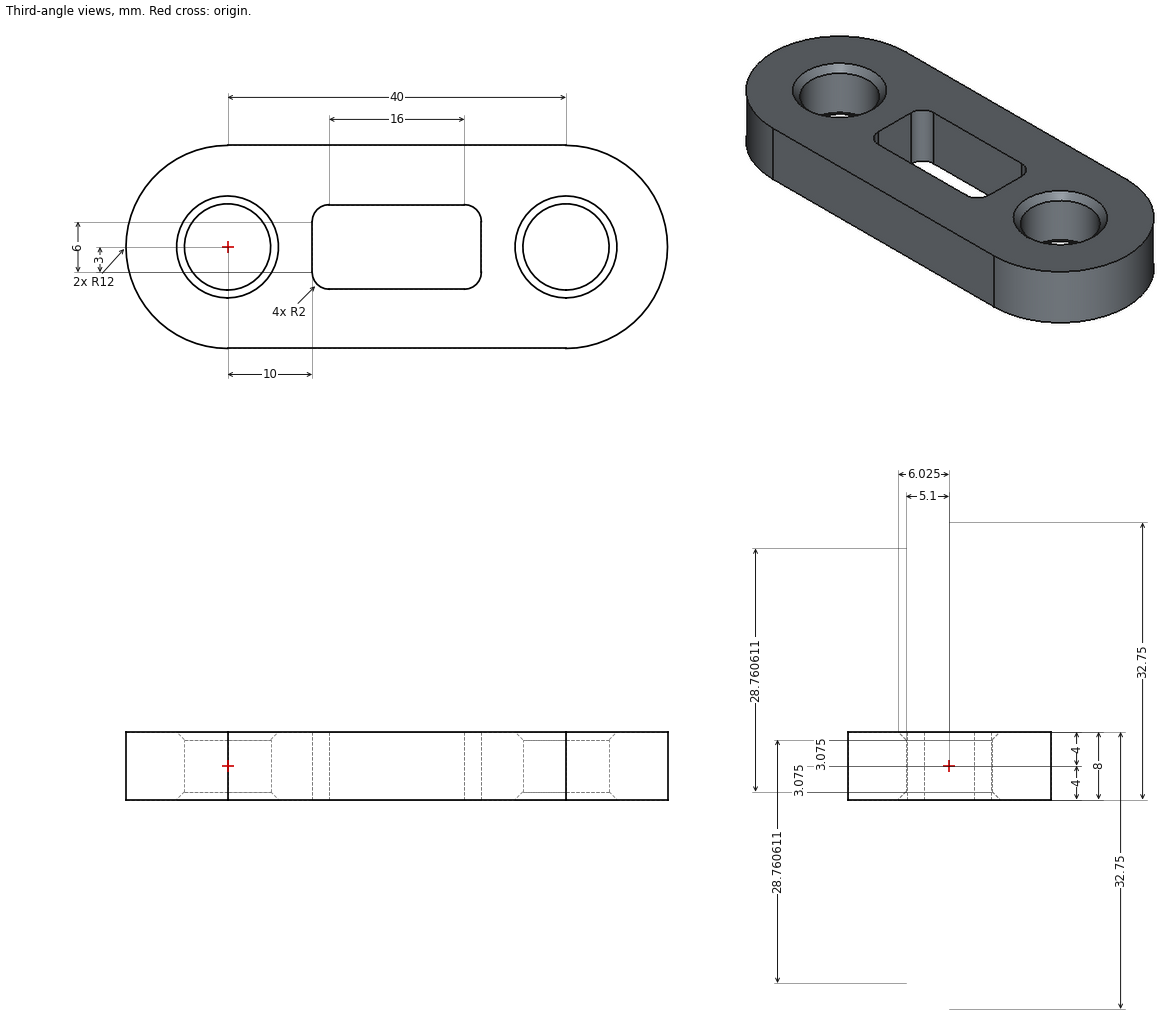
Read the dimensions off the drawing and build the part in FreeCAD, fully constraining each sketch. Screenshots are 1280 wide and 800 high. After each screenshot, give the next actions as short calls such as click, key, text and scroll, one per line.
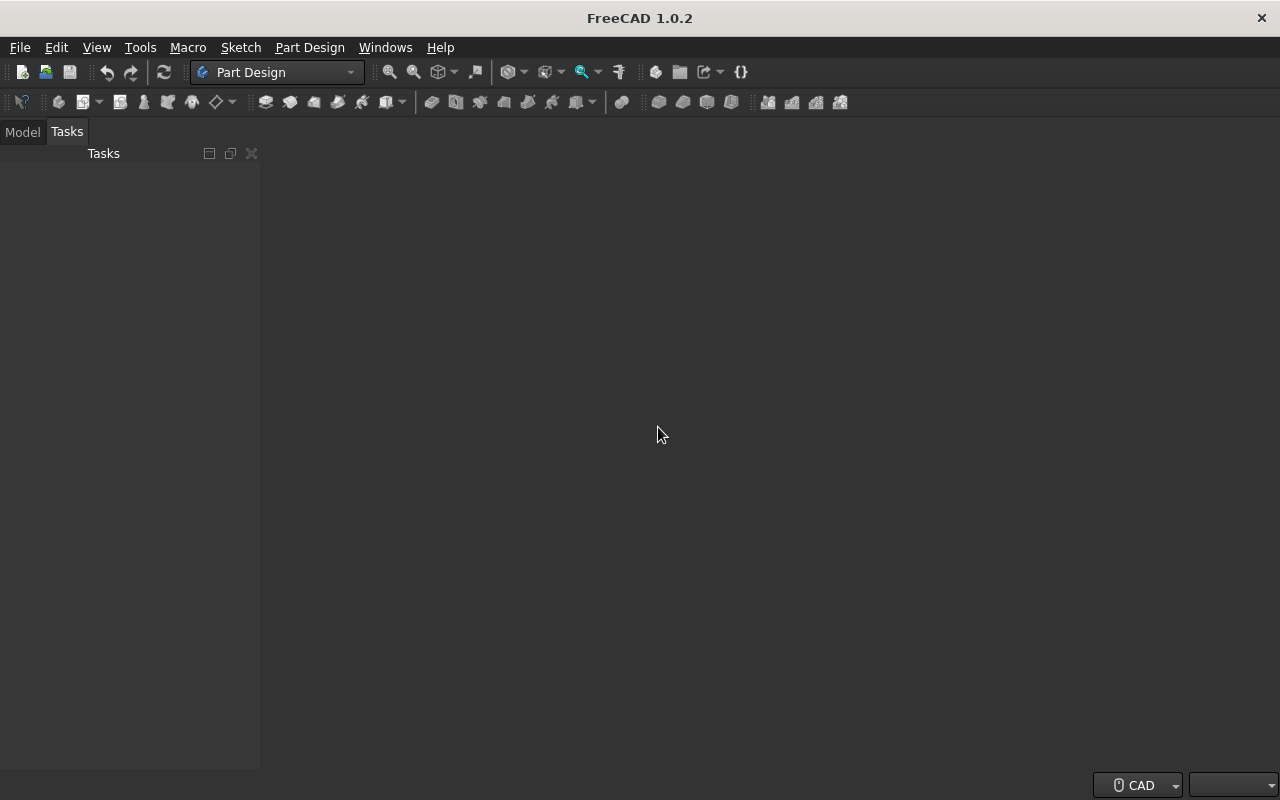
key(ctrl+n)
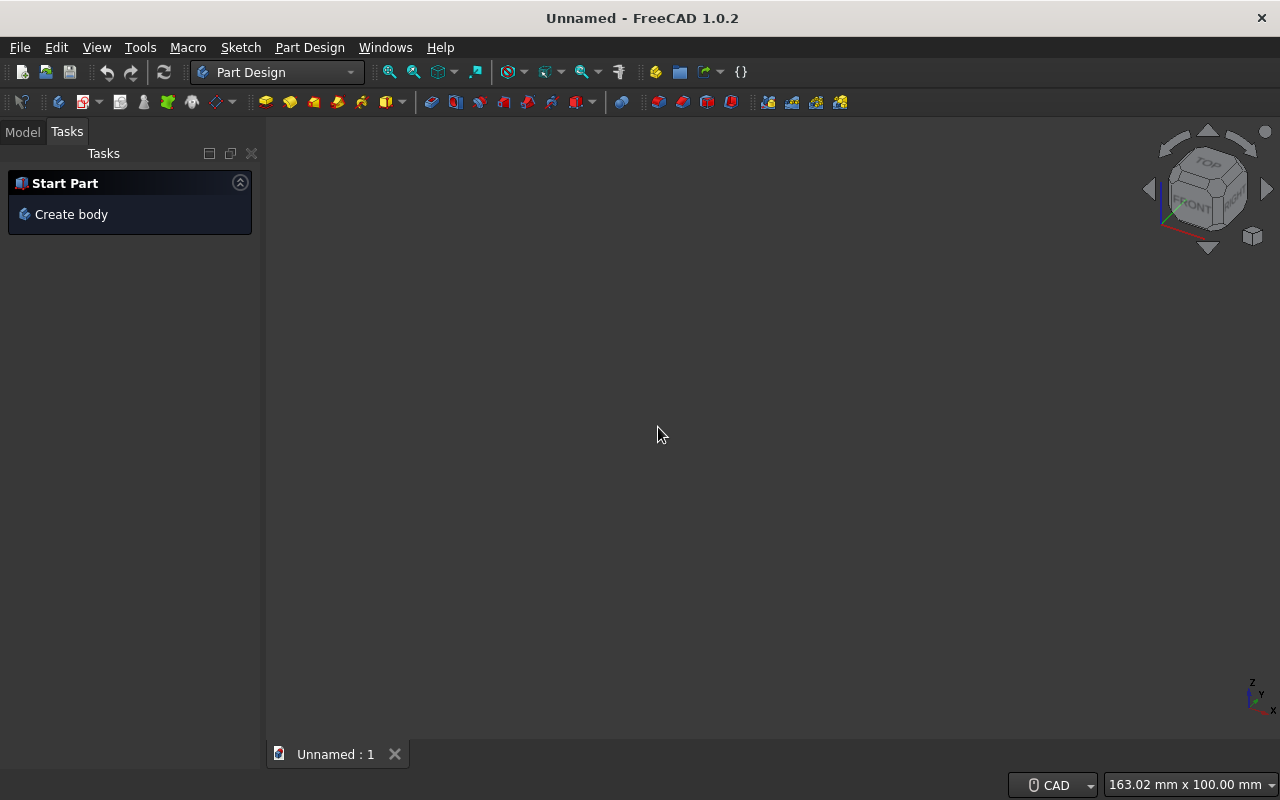
click(84, 102)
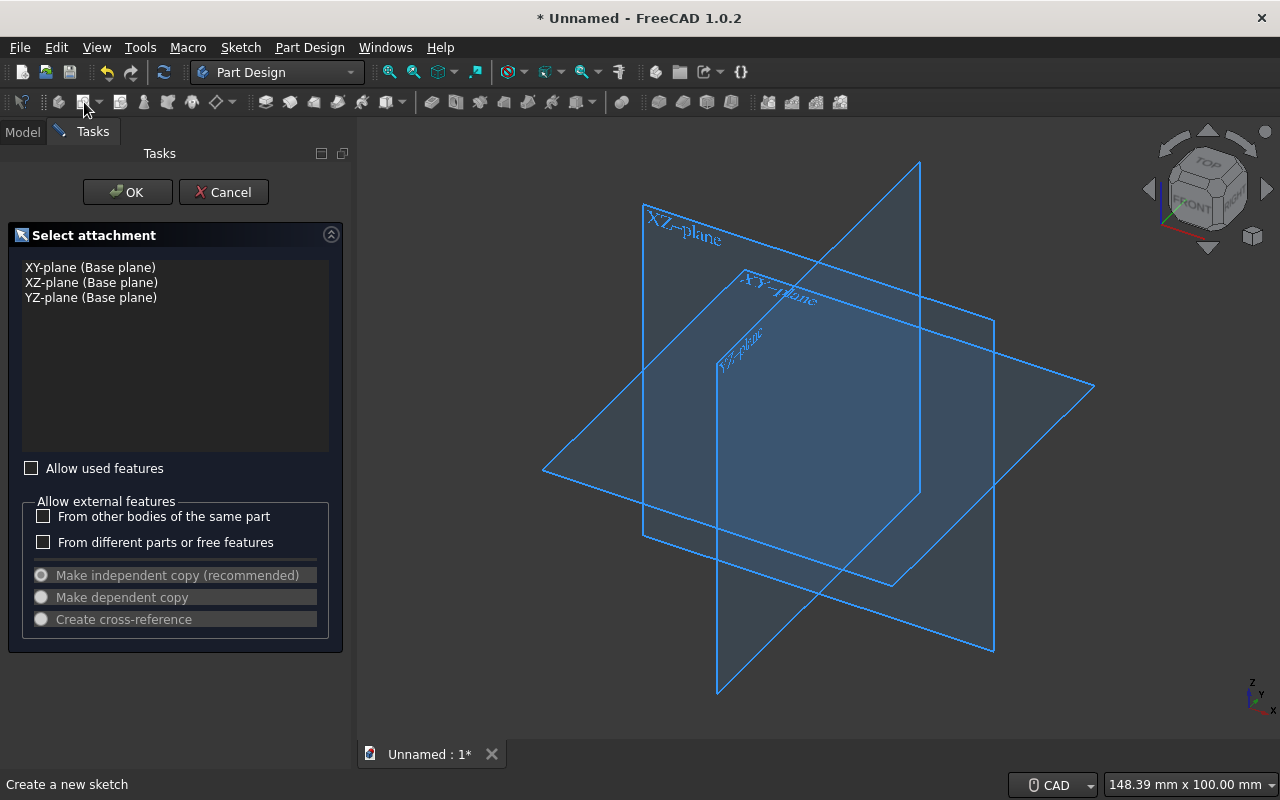
click(82, 268)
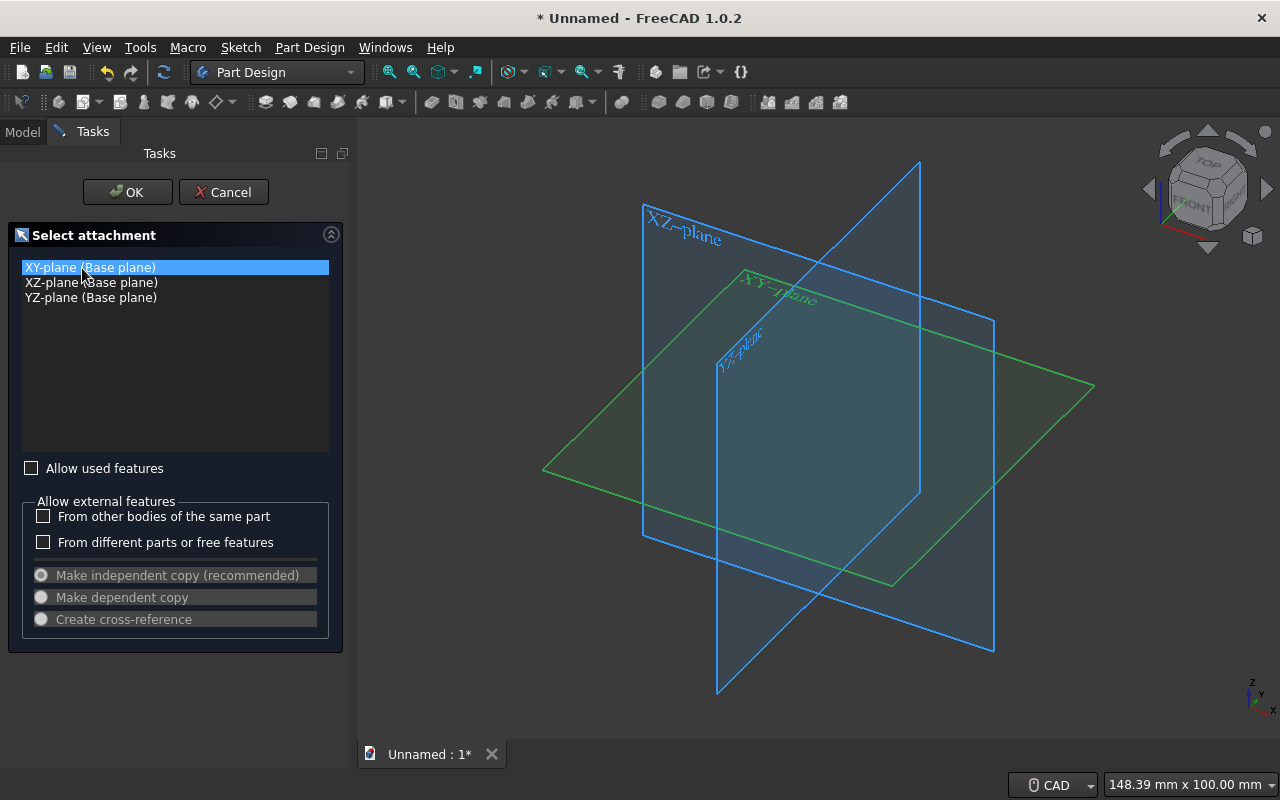
click(128, 192)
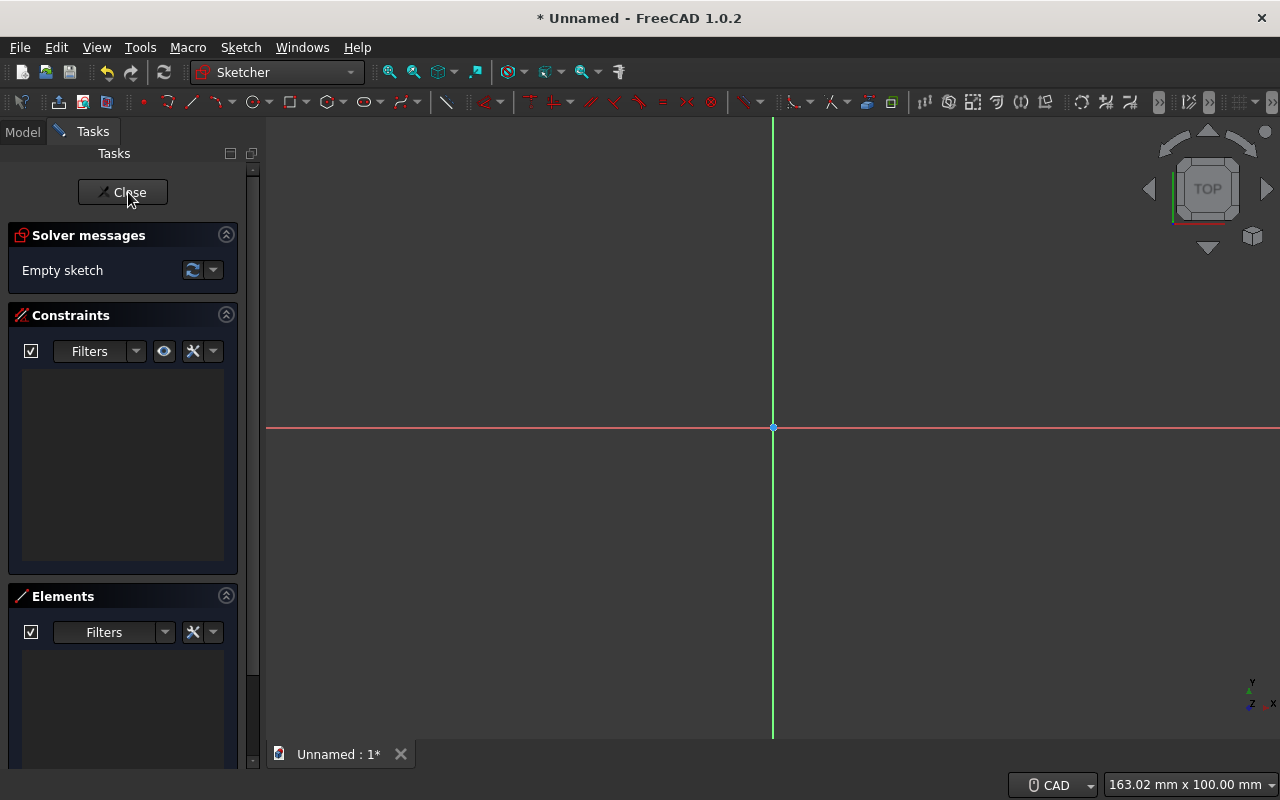
scroll(1115, 428, up, 2)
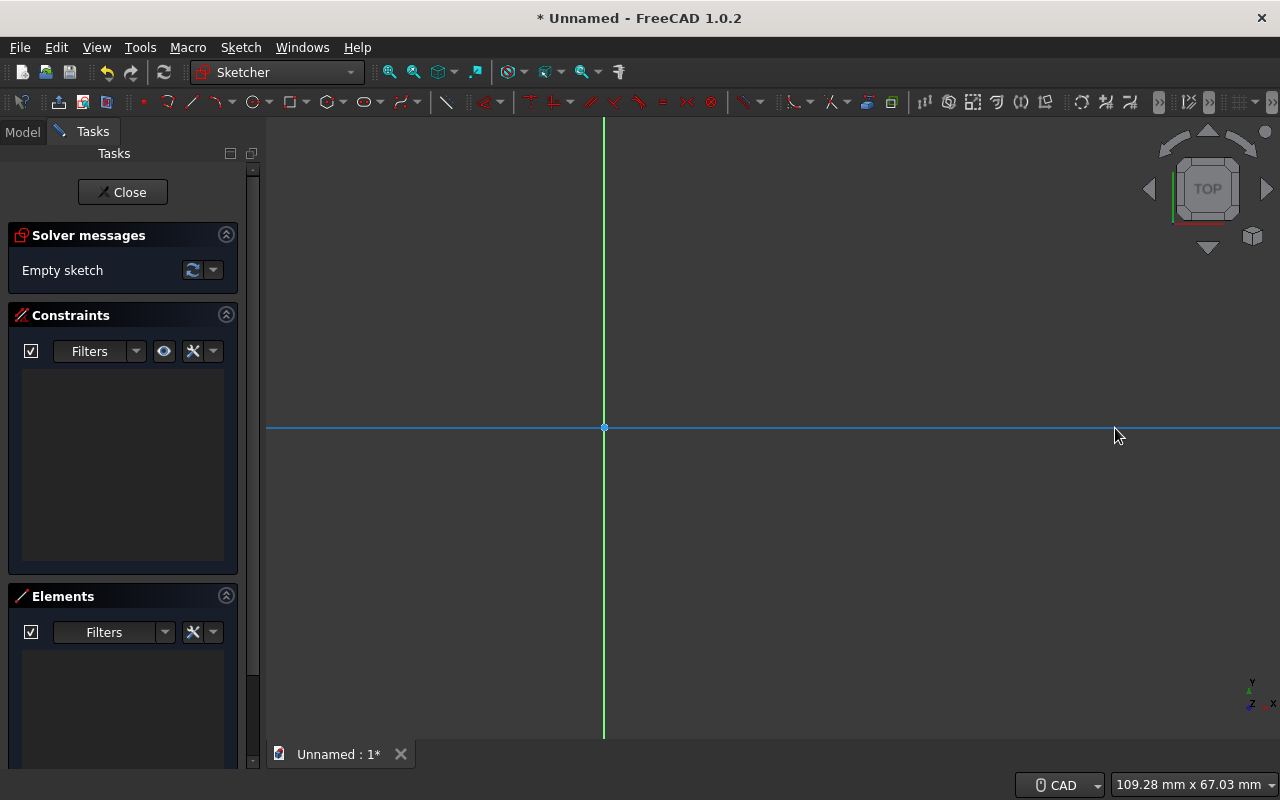
key(g)
key(s)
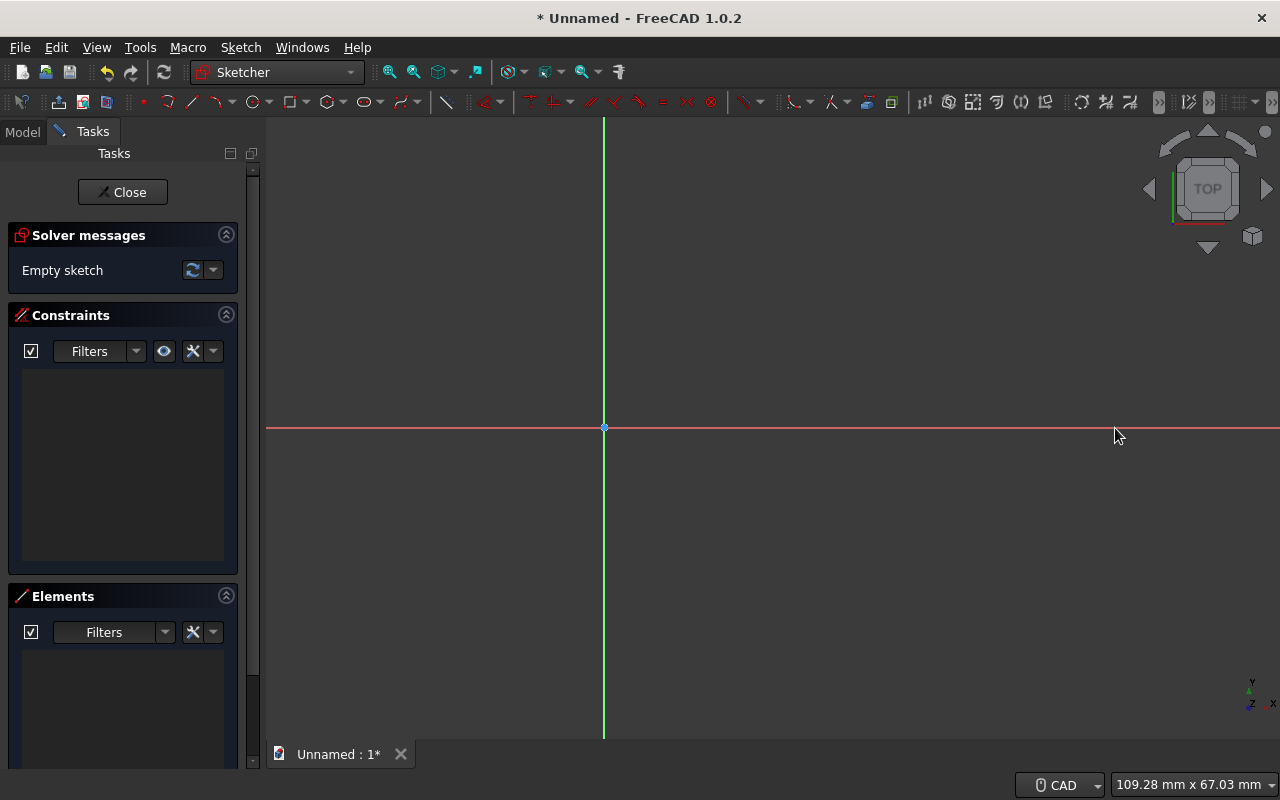
click(604, 428)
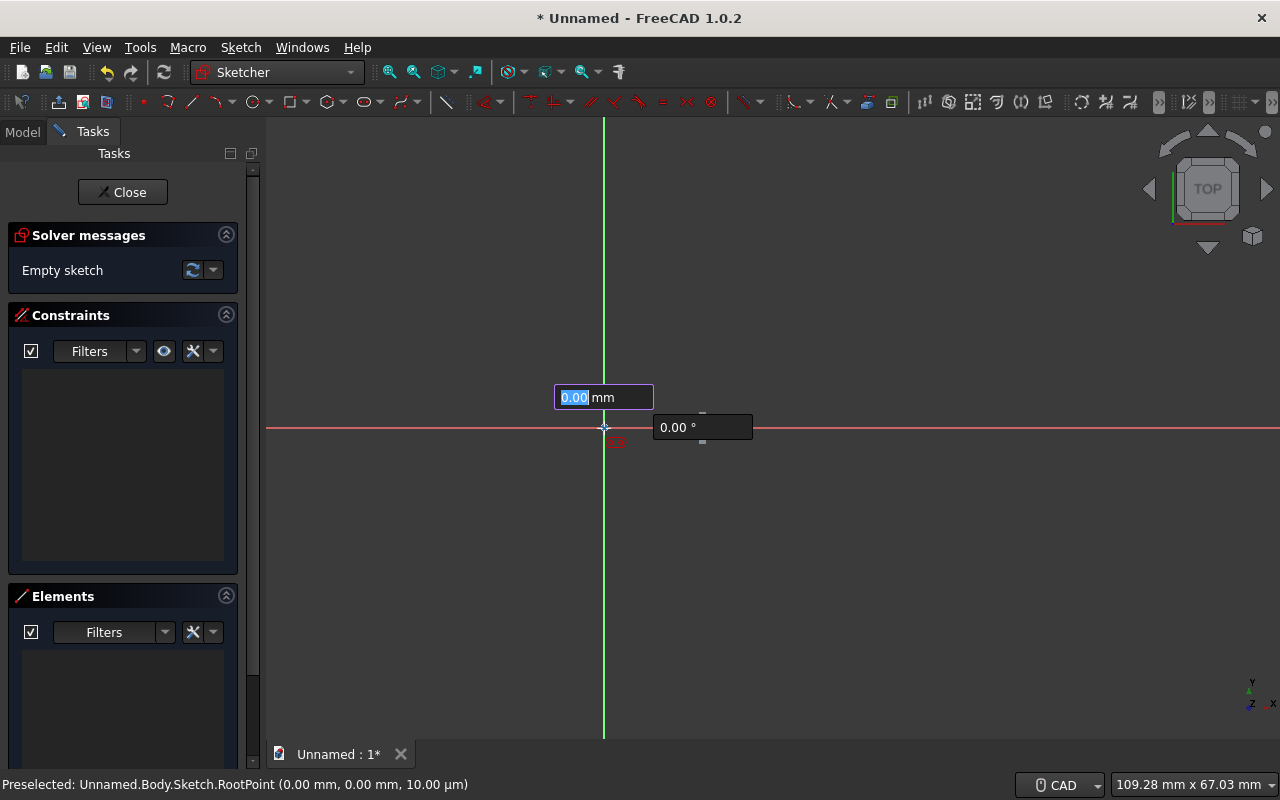
click(976, 419)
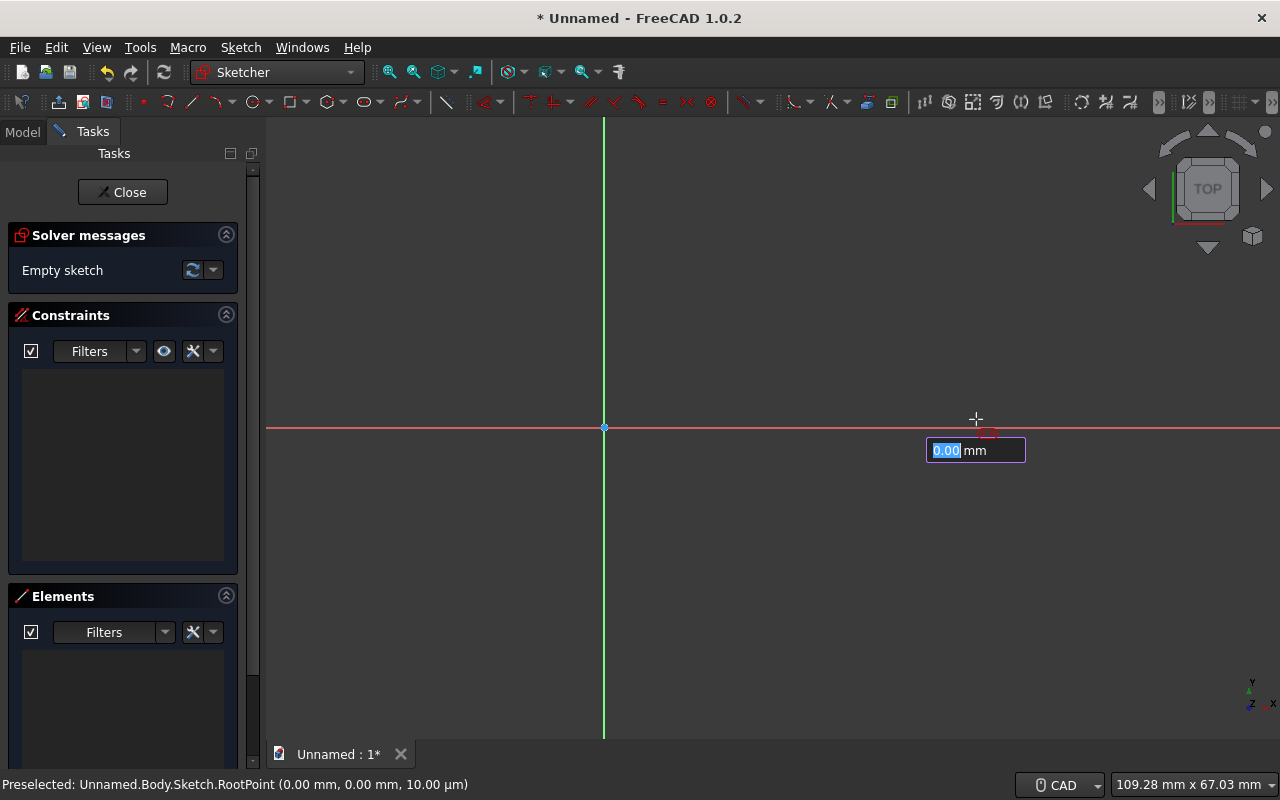
click(790, 316)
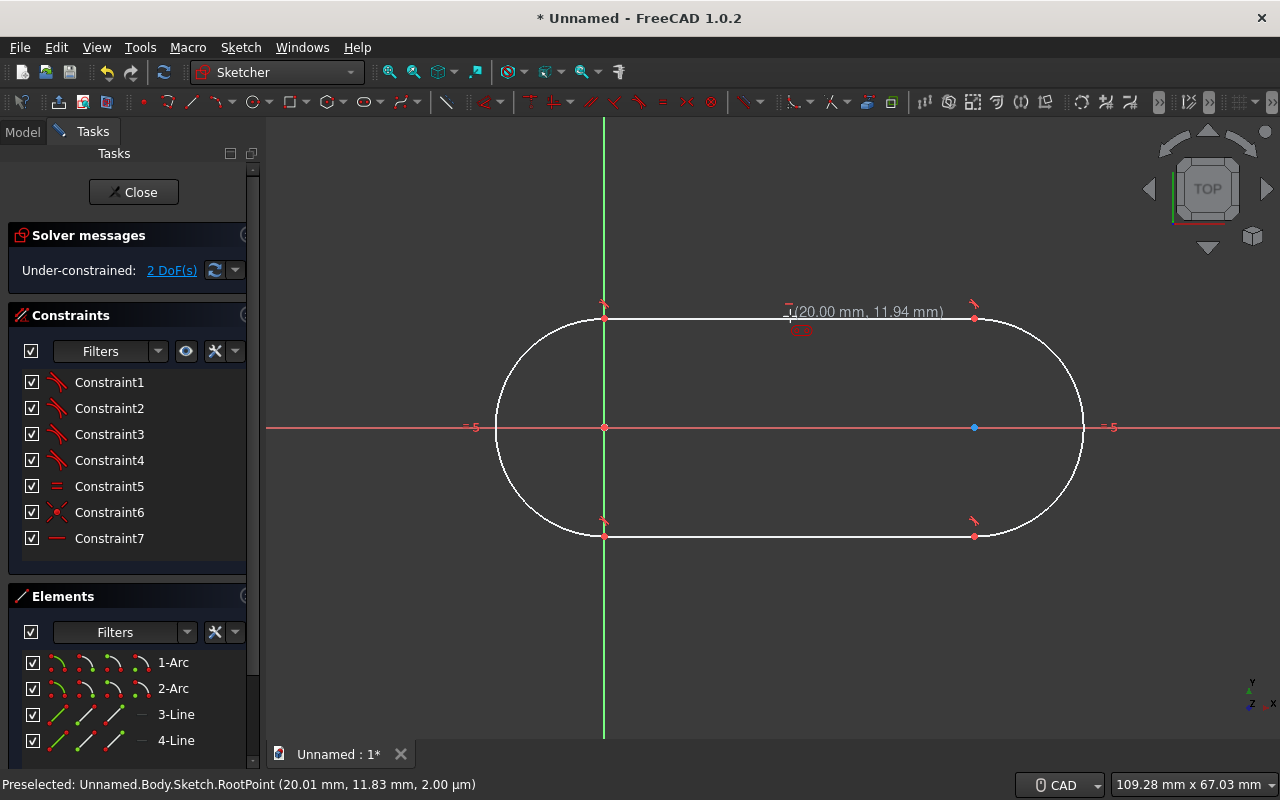
key(g)
key(l)